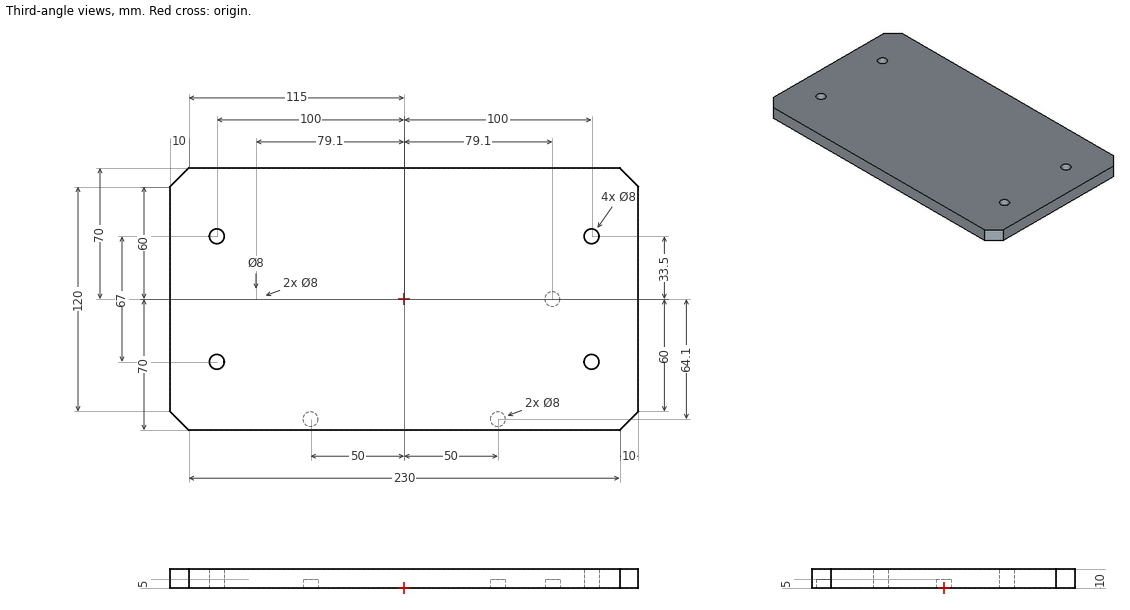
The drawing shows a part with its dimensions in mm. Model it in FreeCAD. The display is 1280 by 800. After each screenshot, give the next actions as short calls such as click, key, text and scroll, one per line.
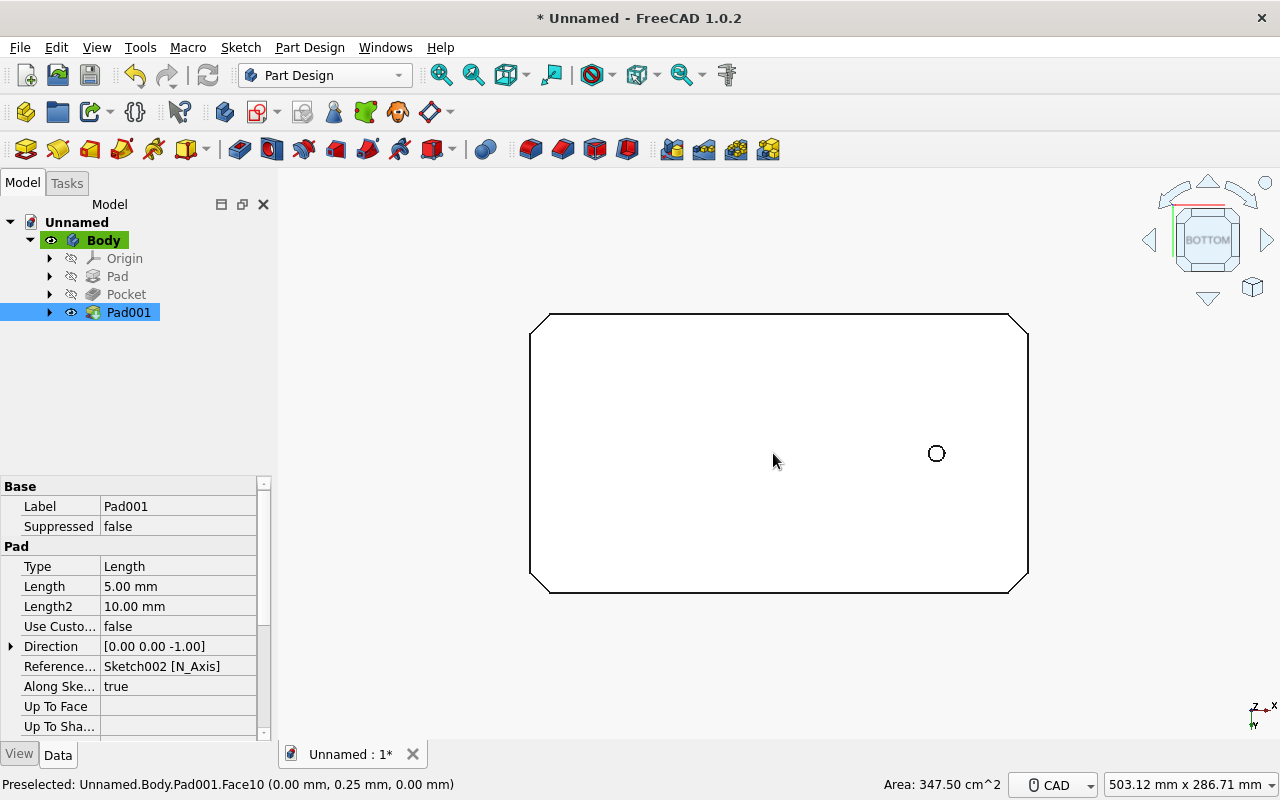
click(258, 112)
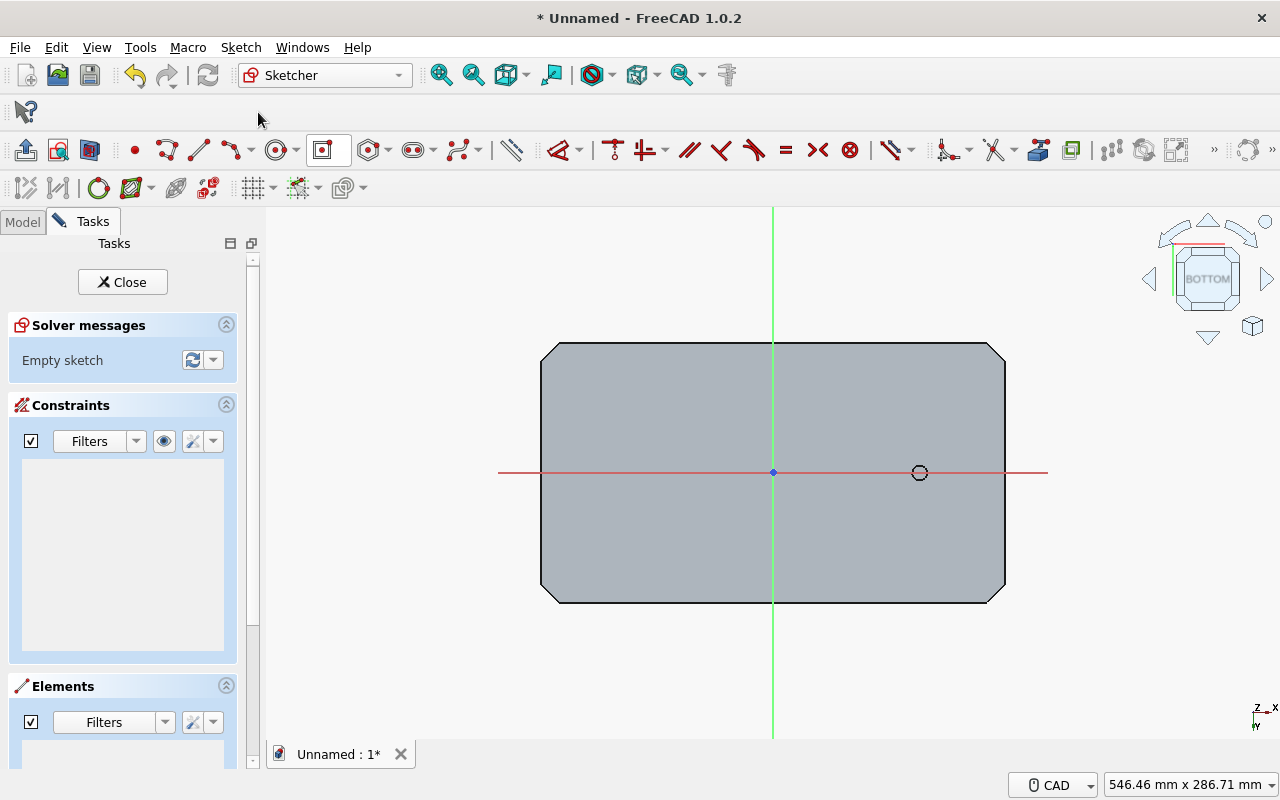
scroll(813, 373, up, 5)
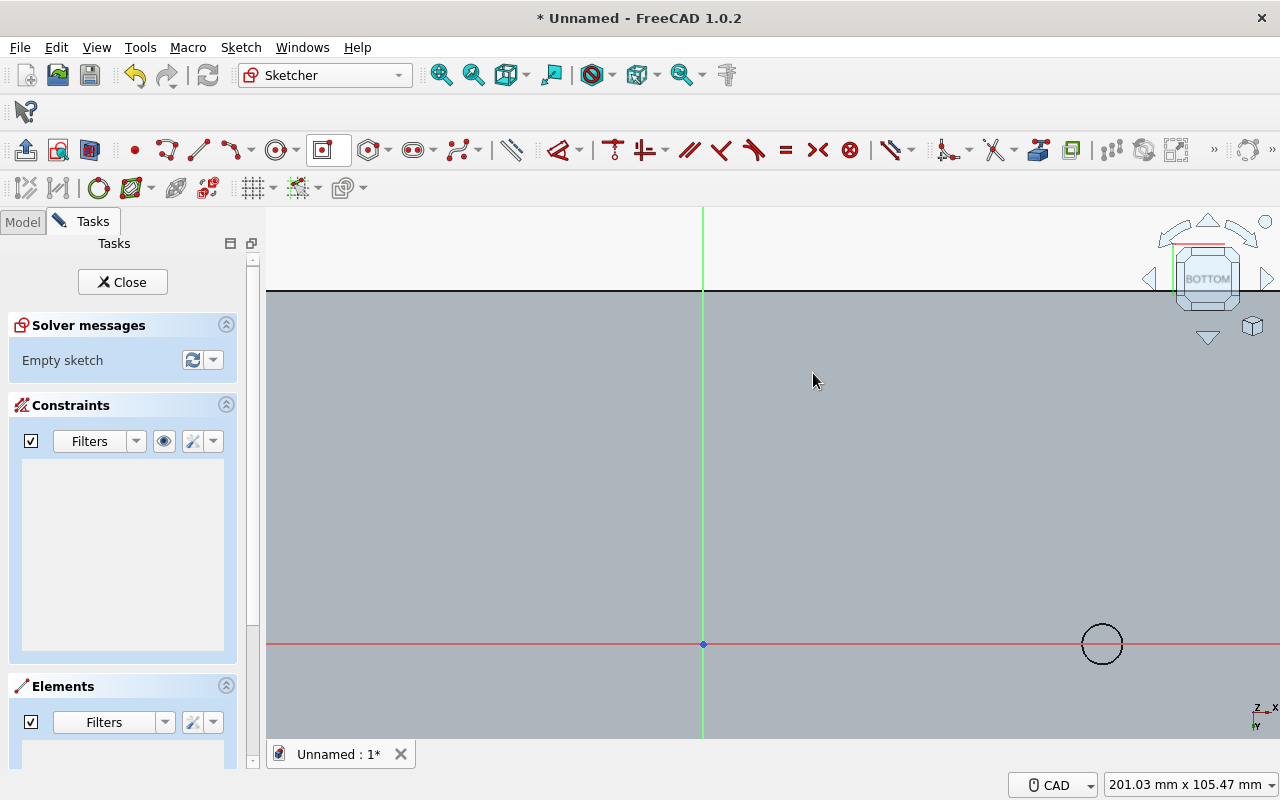
click(276, 150)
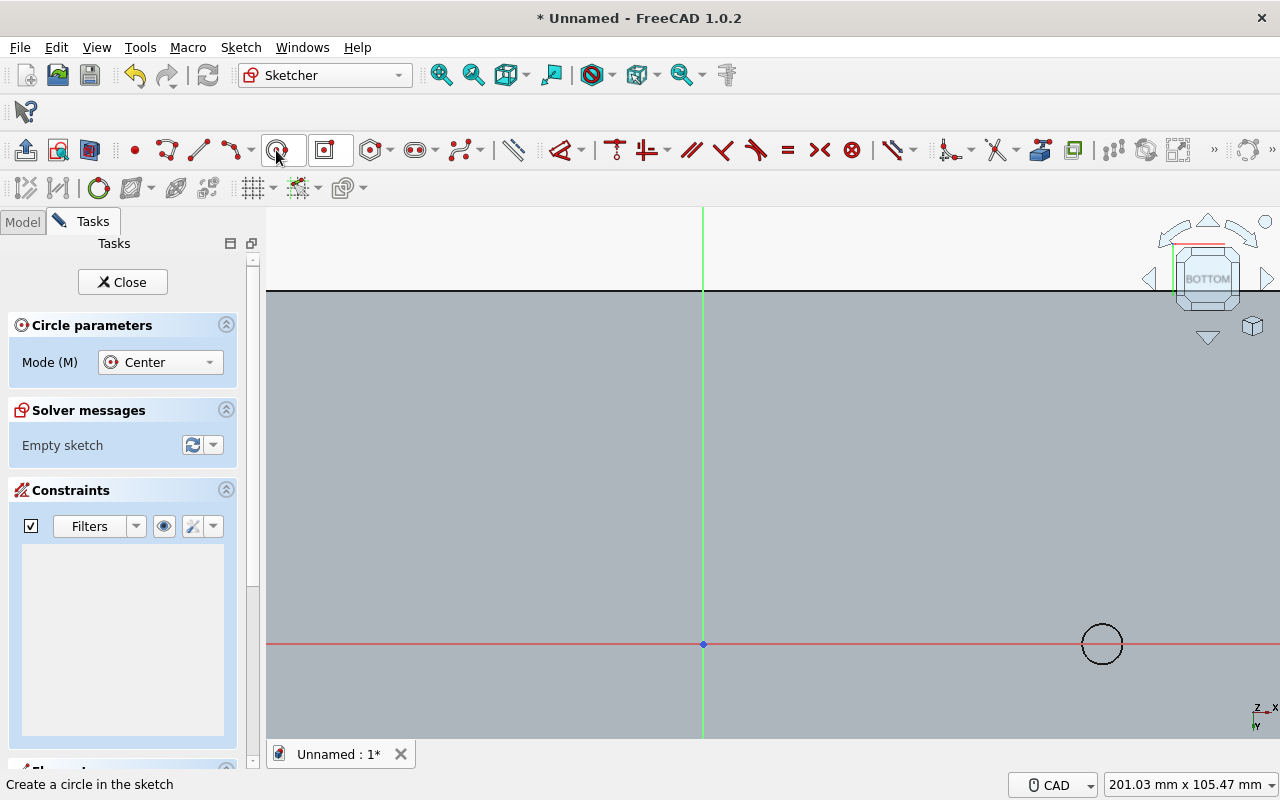
click(956, 321)
click(970, 307)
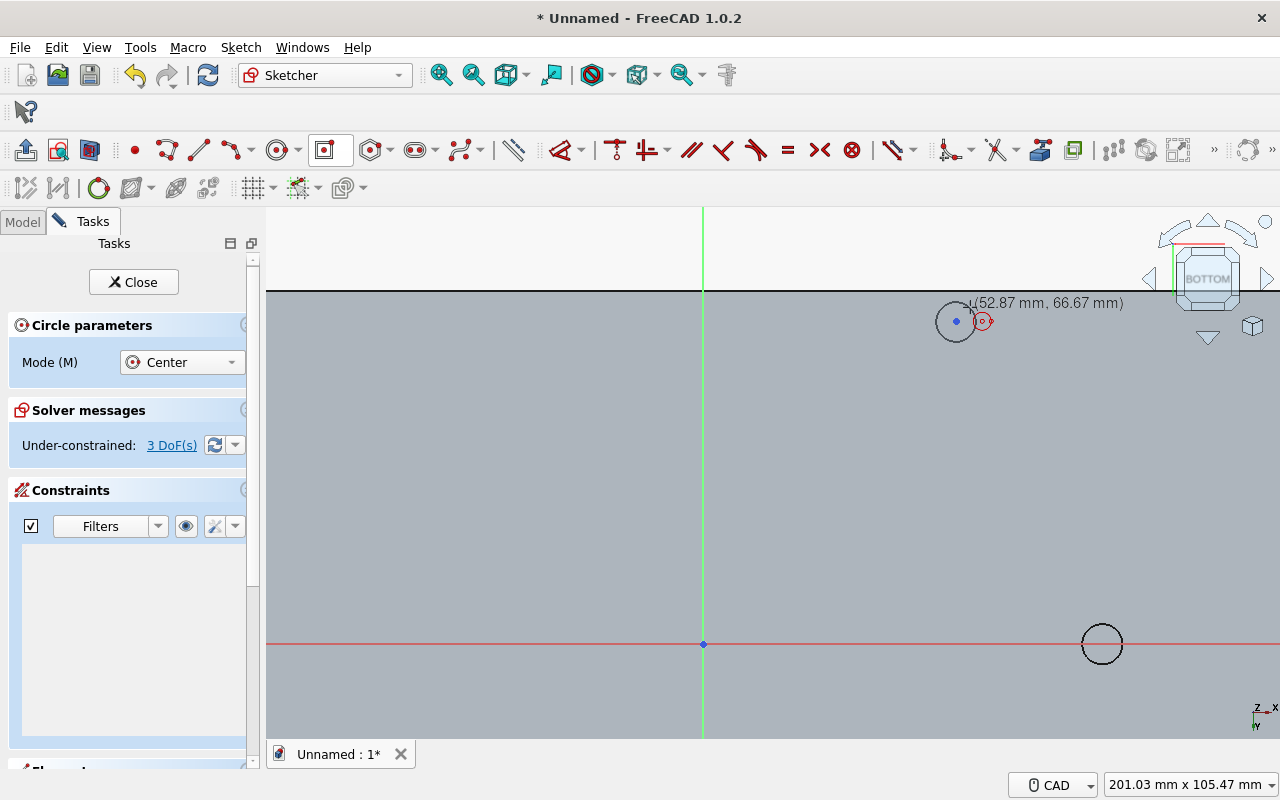
click(451, 321)
click(465, 307)
key(Escape)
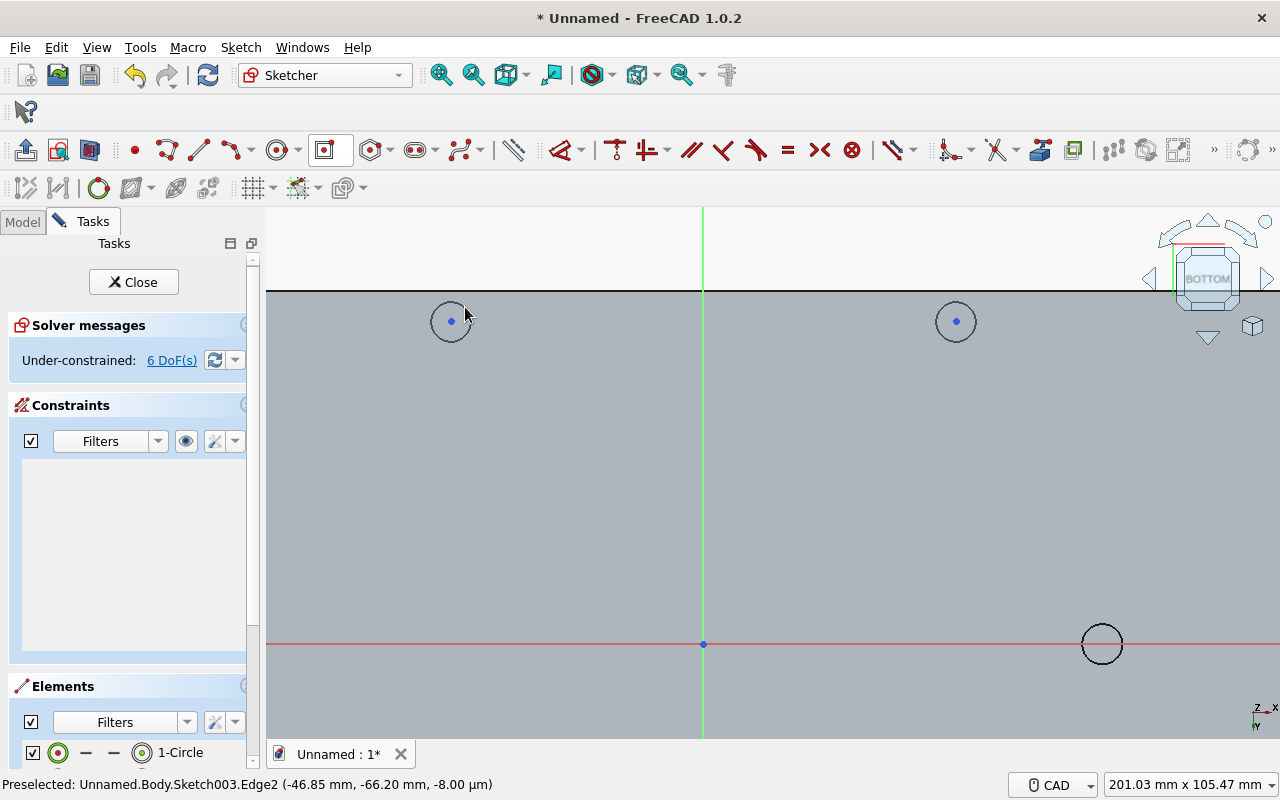
click(970, 308)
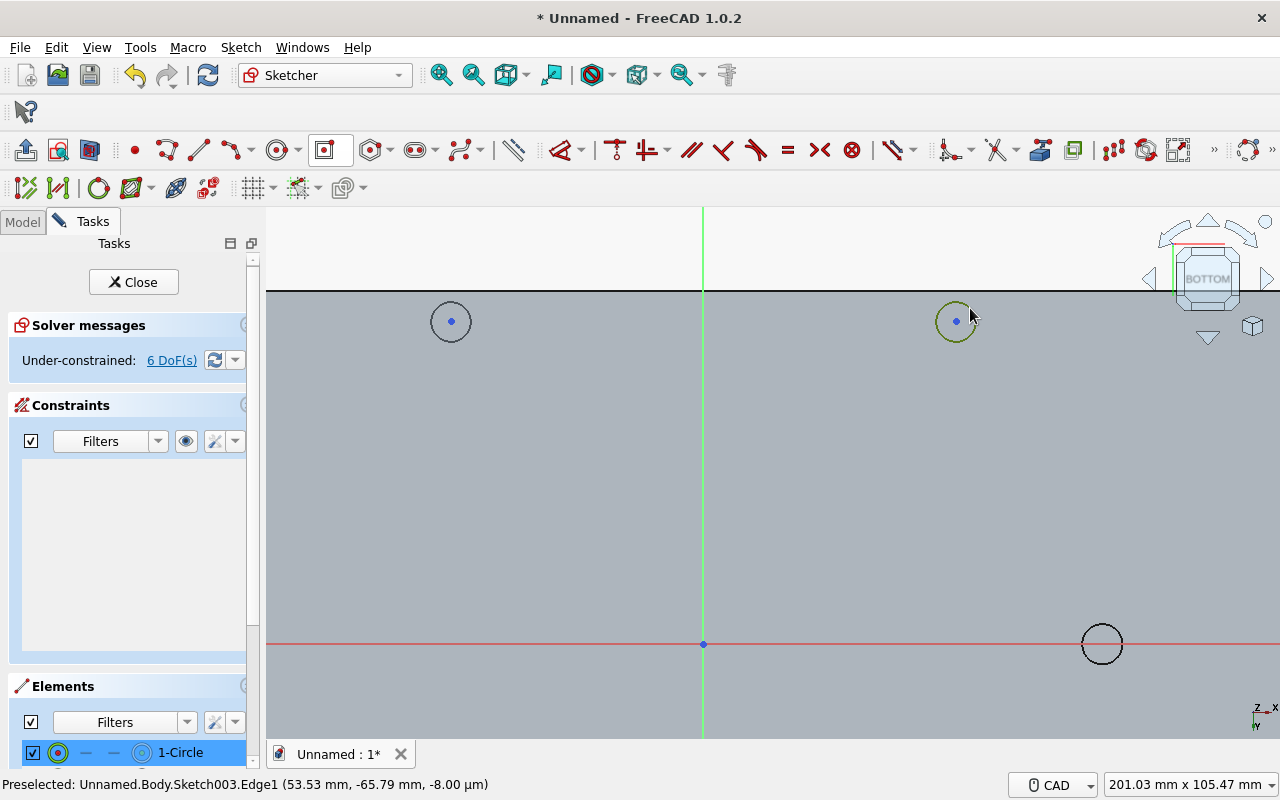
click(465, 308)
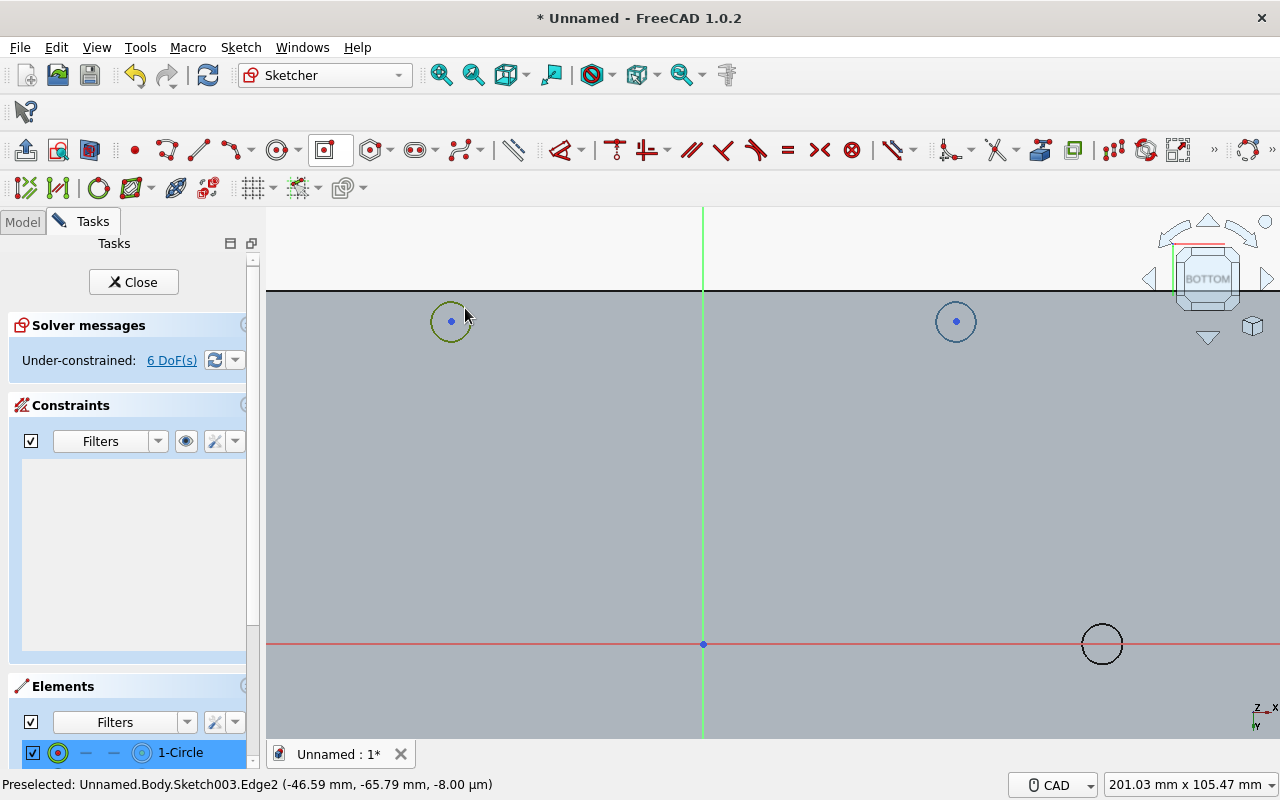
click(788, 150)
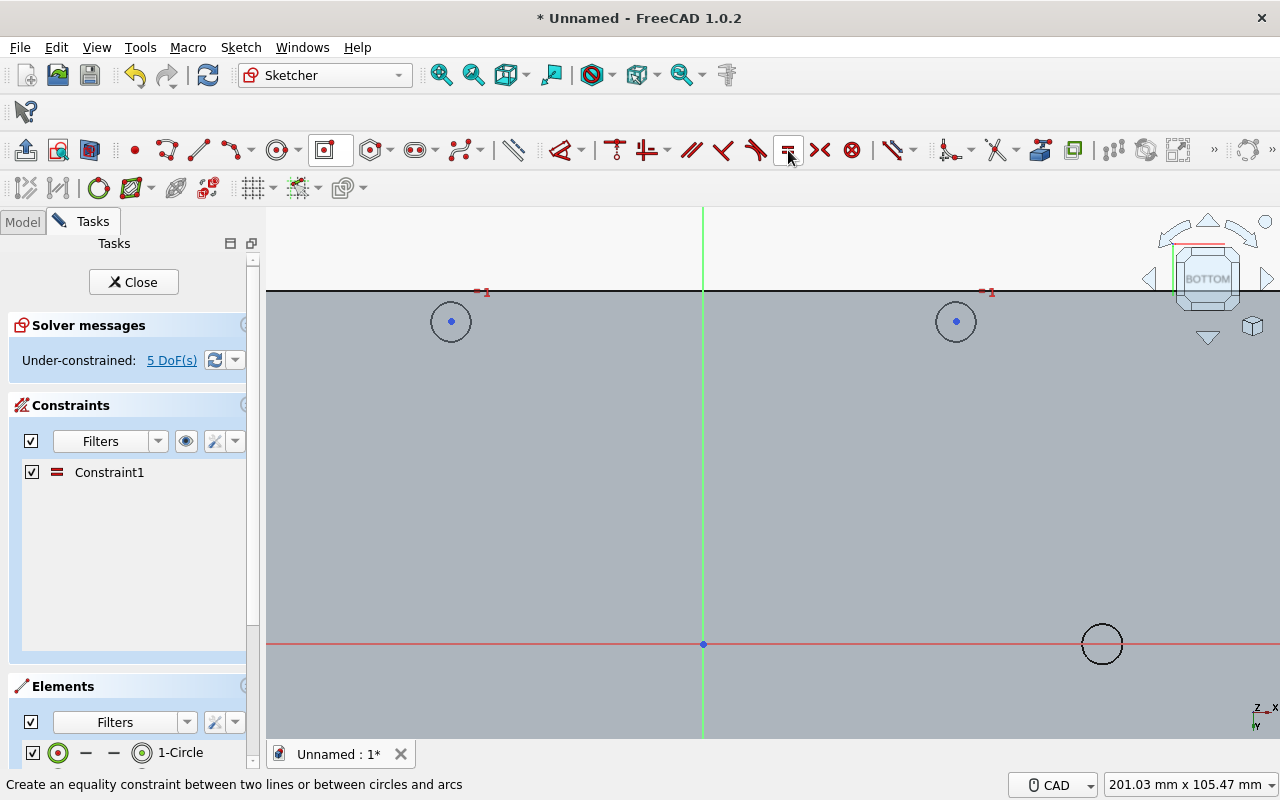
click(956, 322)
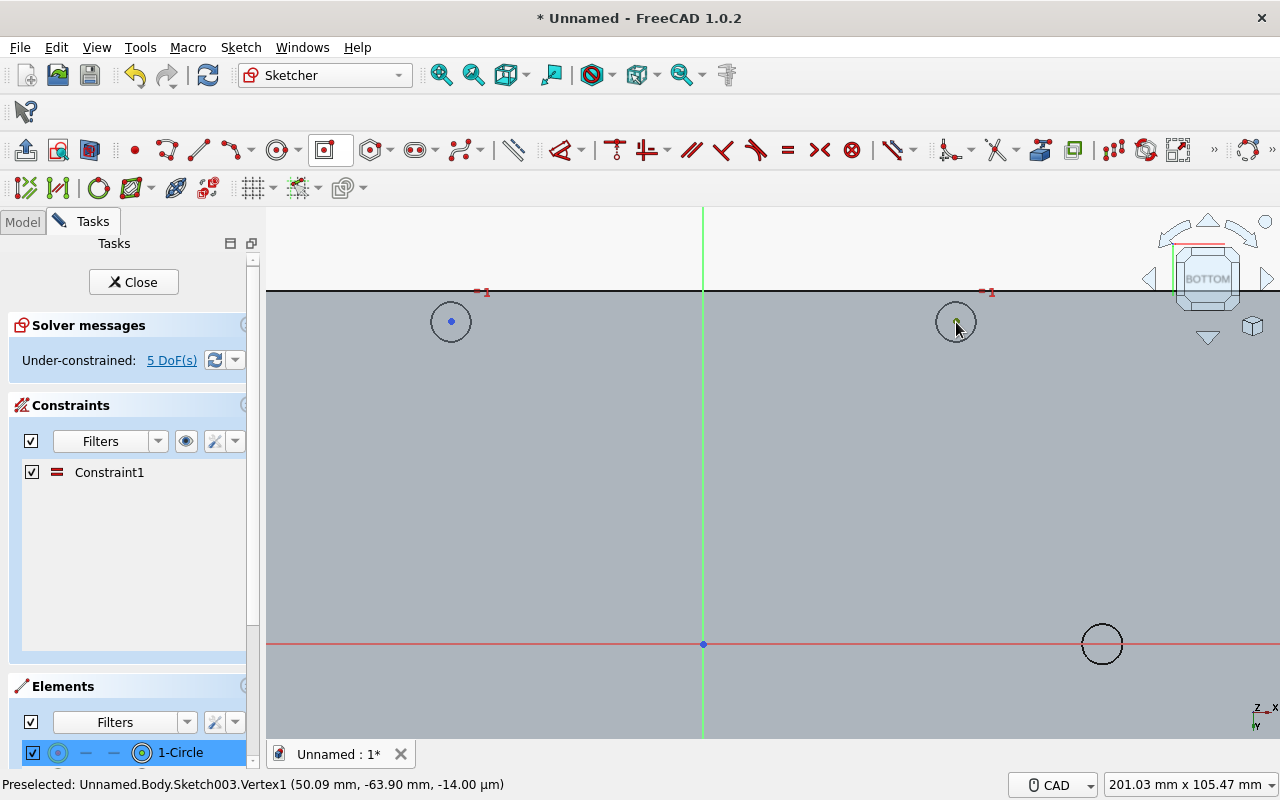
click(451, 322)